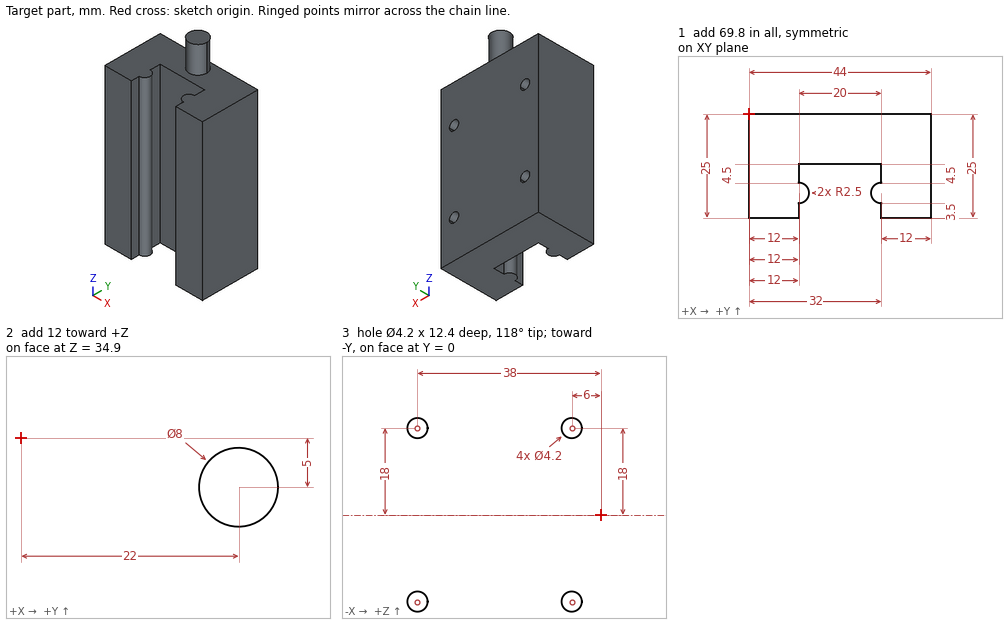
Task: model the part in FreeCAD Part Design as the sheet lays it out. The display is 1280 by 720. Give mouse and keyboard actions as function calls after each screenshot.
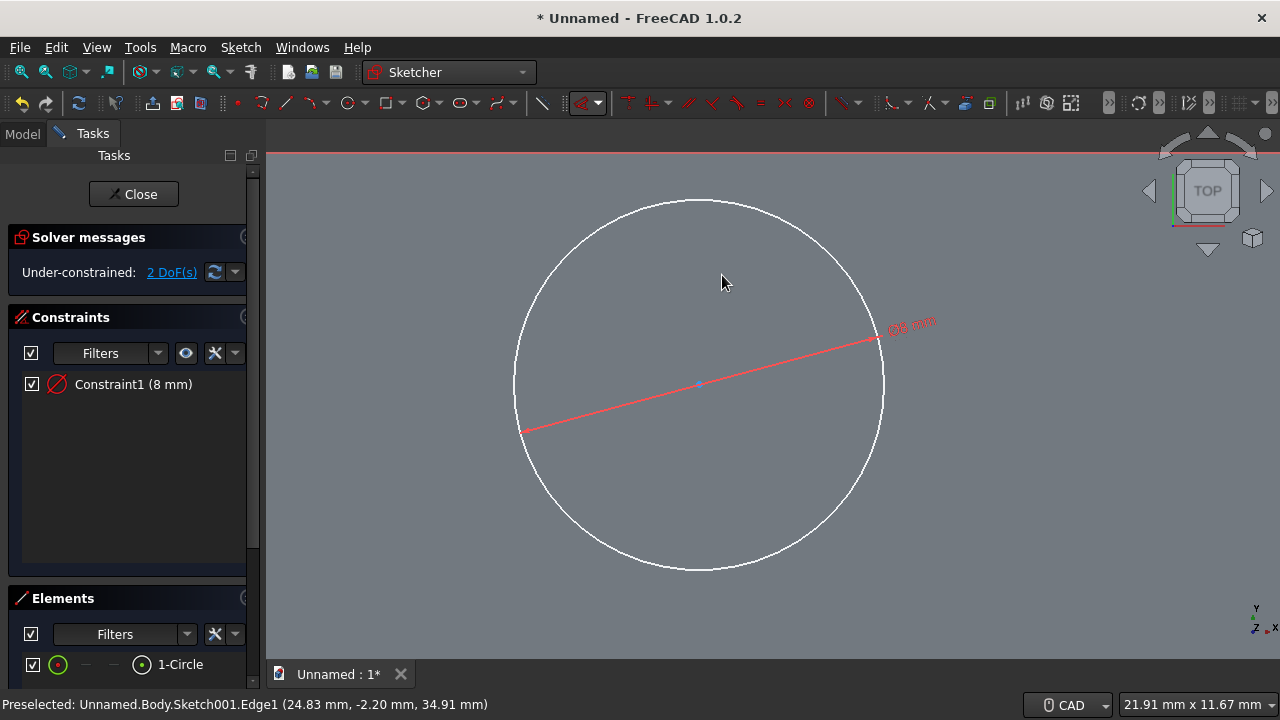
click(699, 385)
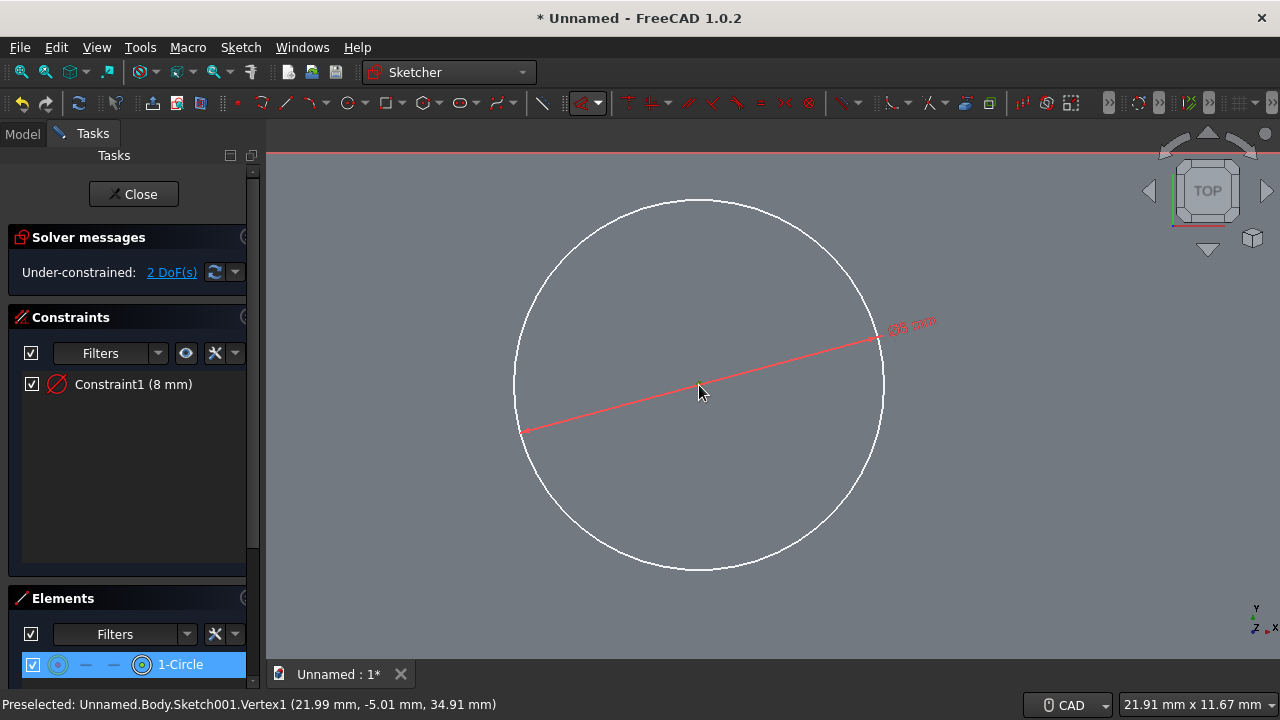
click(600, 104)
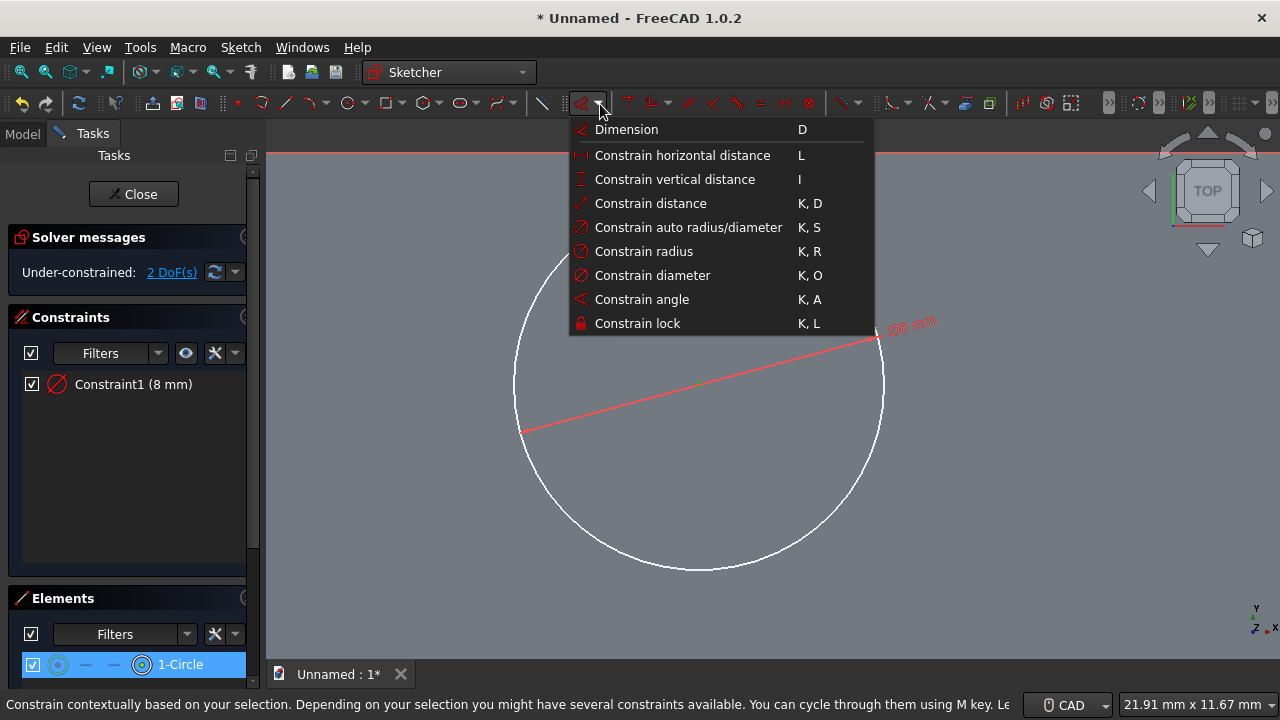
click(722, 179)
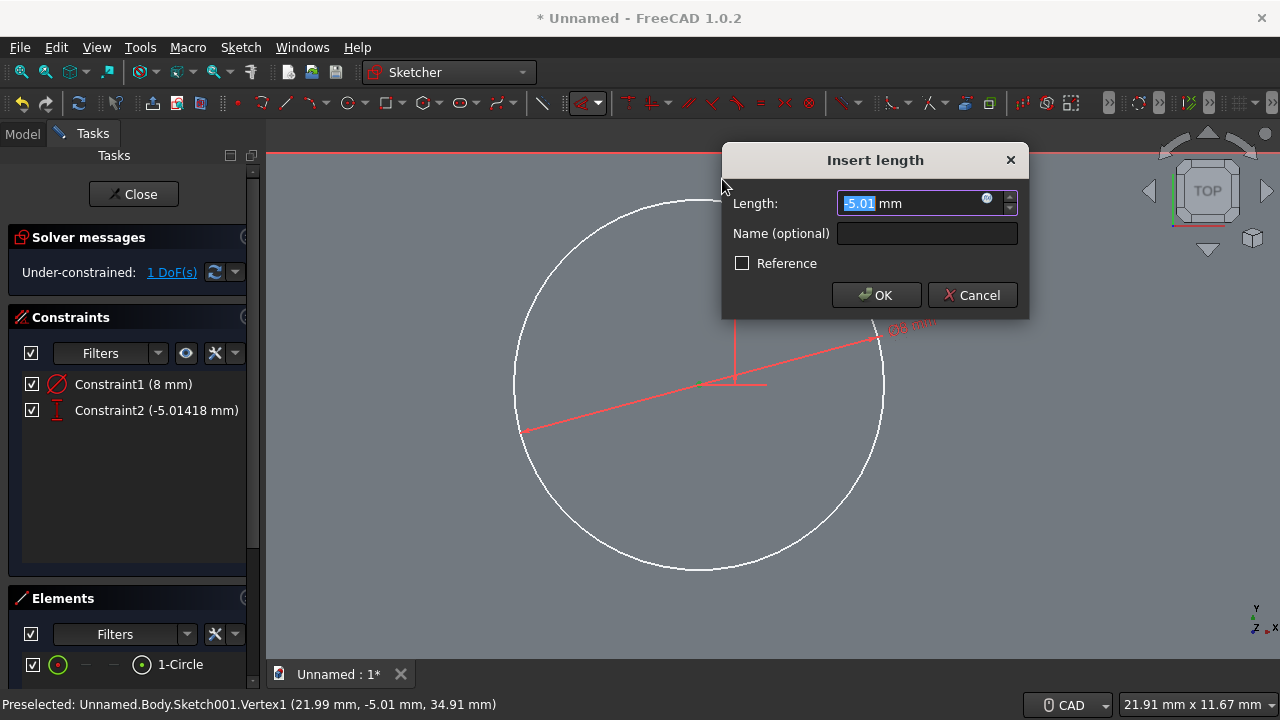
text(-5)
key(Return)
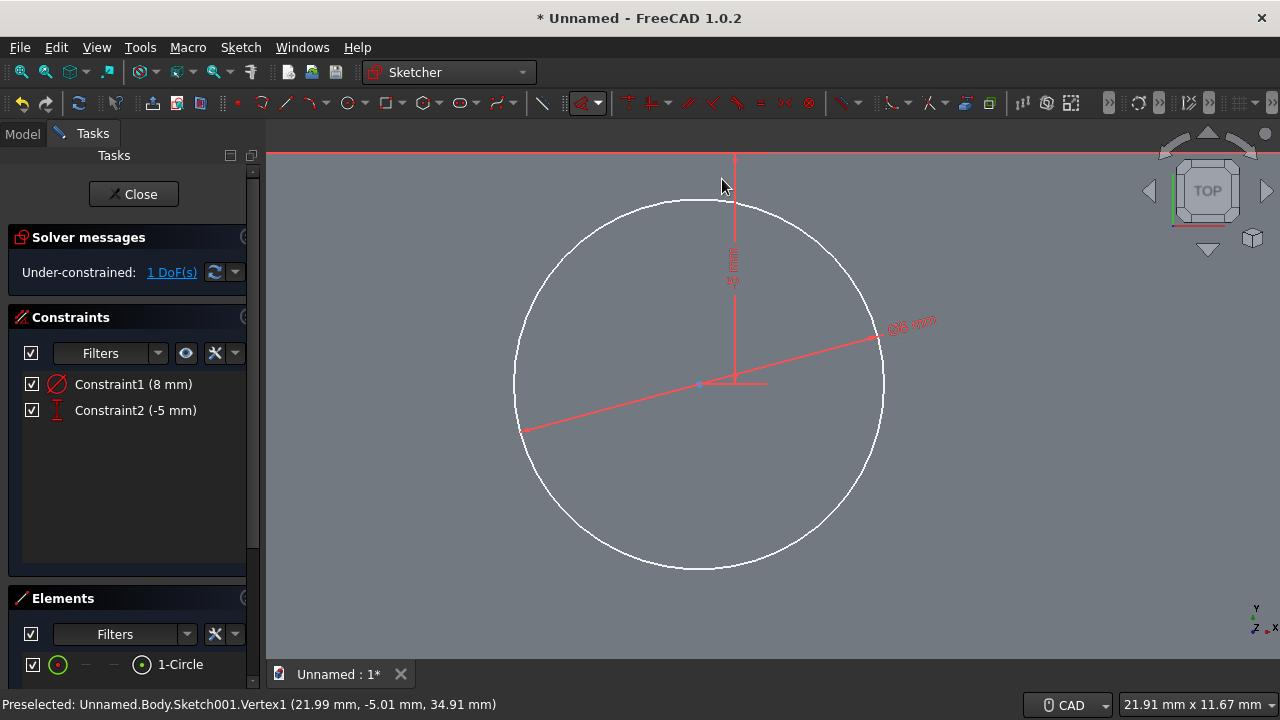
click(699, 384)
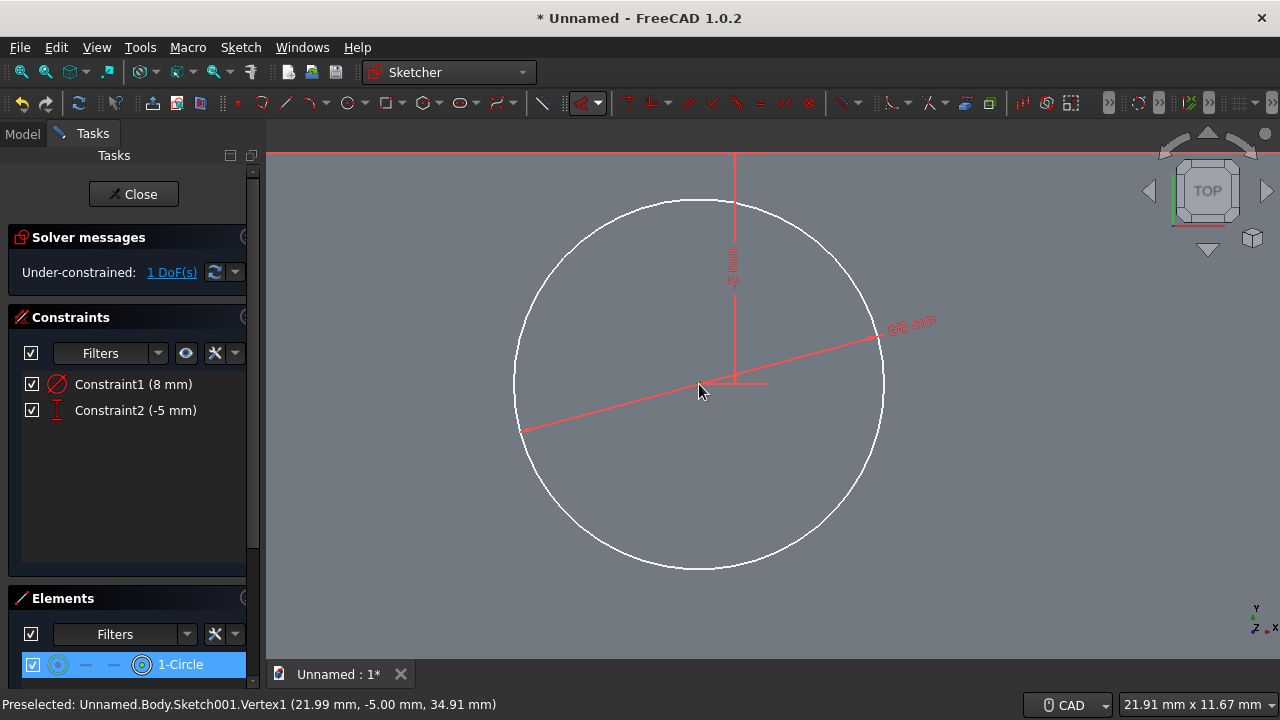
click(600, 104)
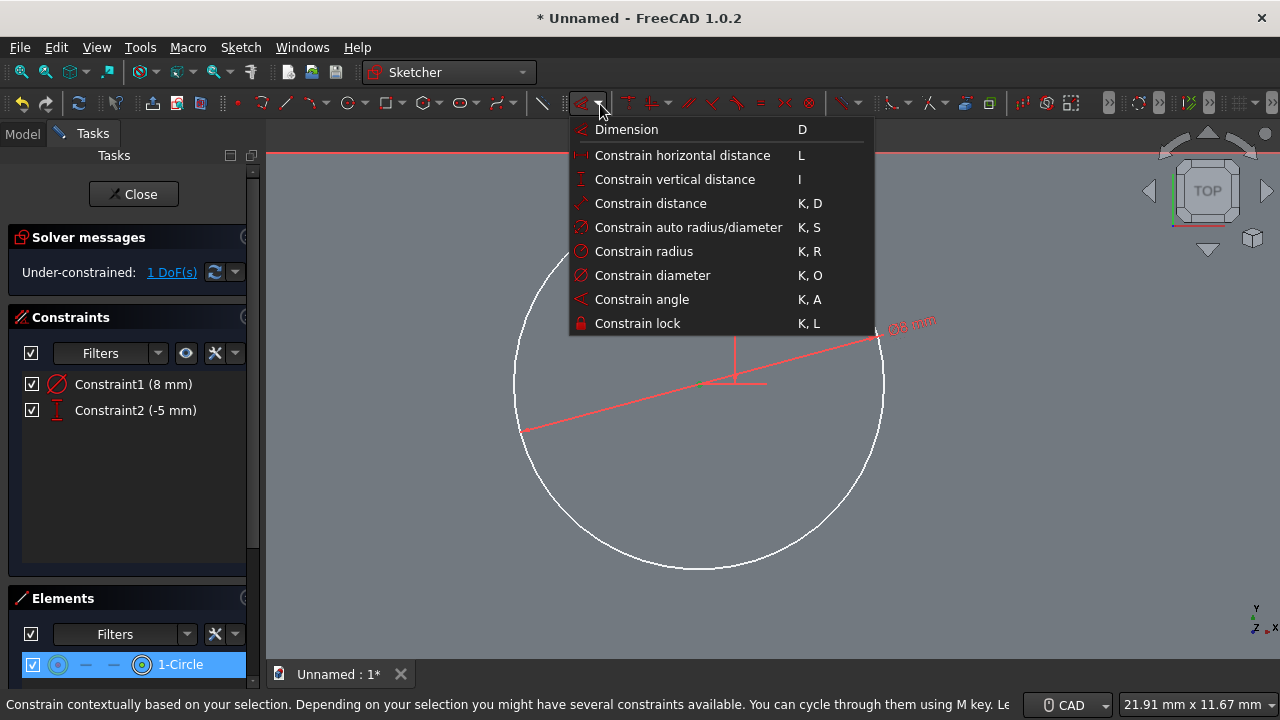
click(722, 155)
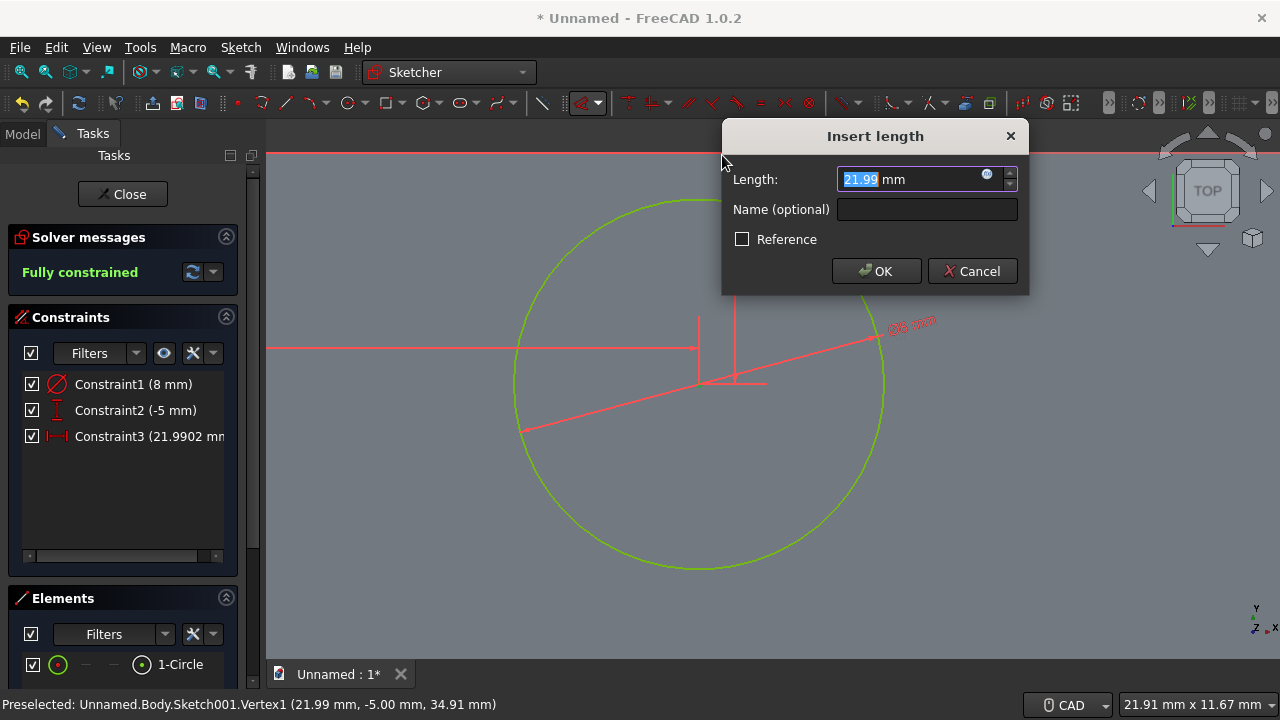
text(22)
key(Return)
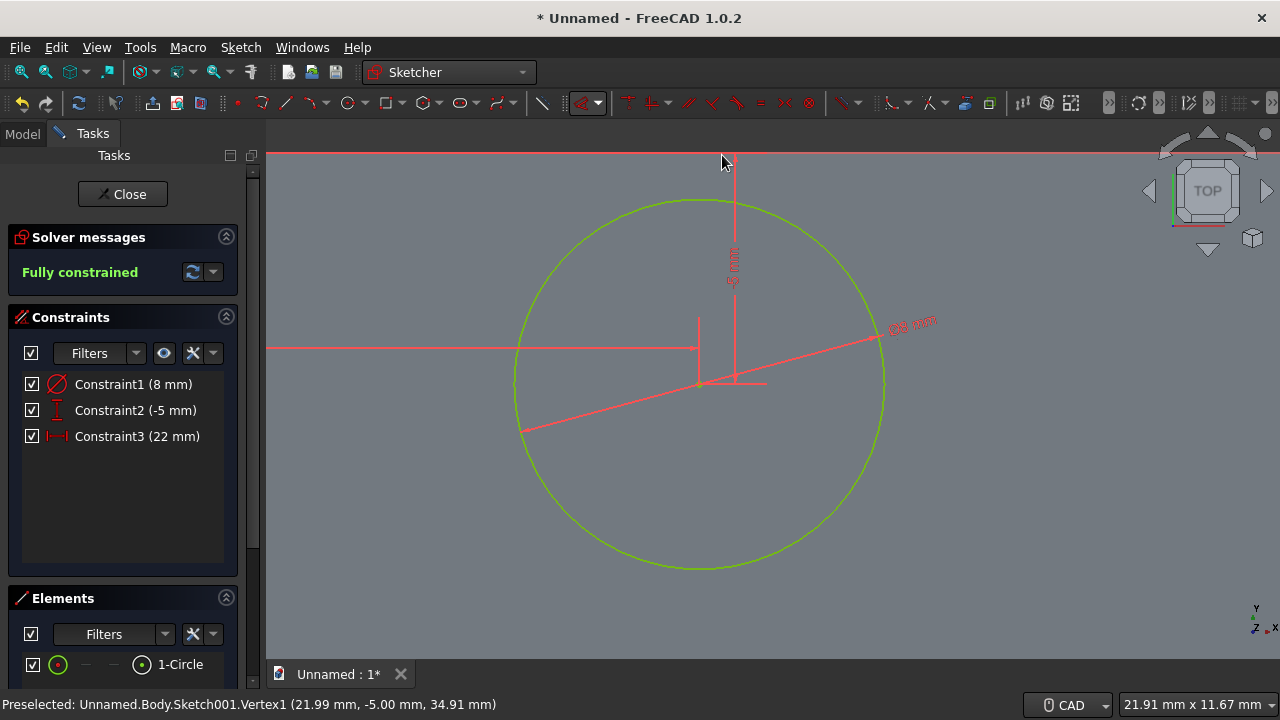
click(123, 194)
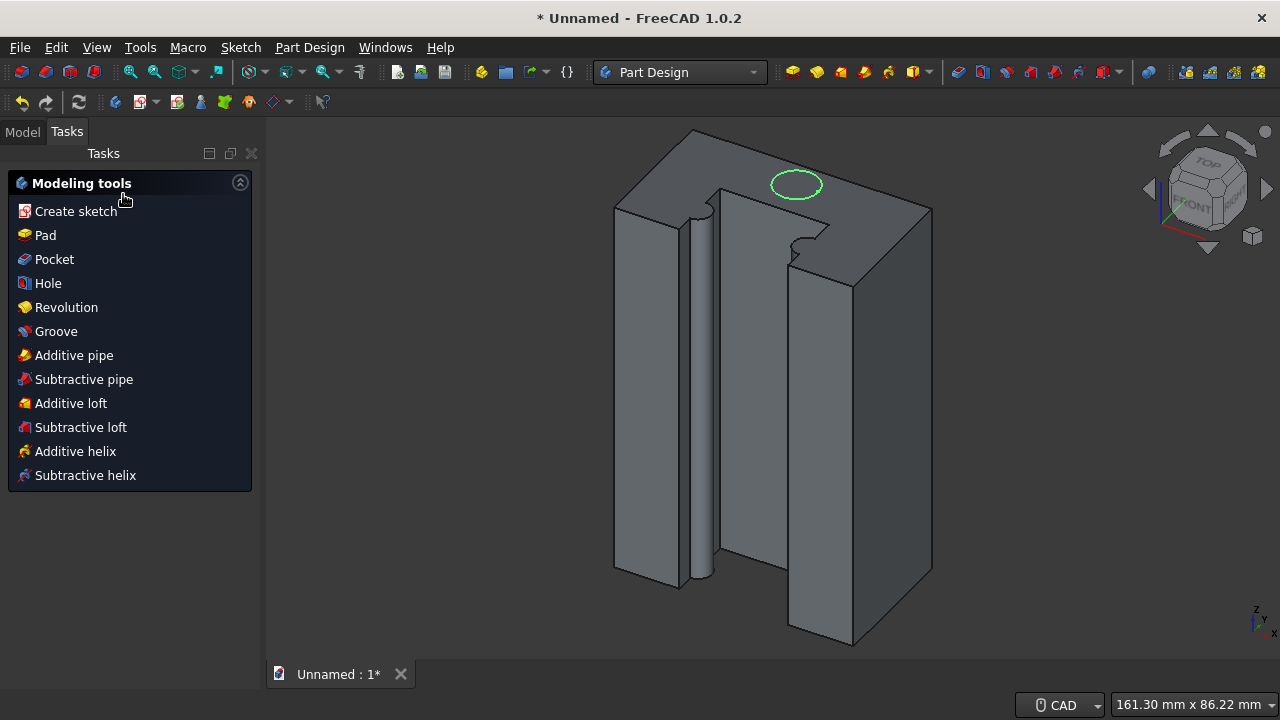
click(794, 72)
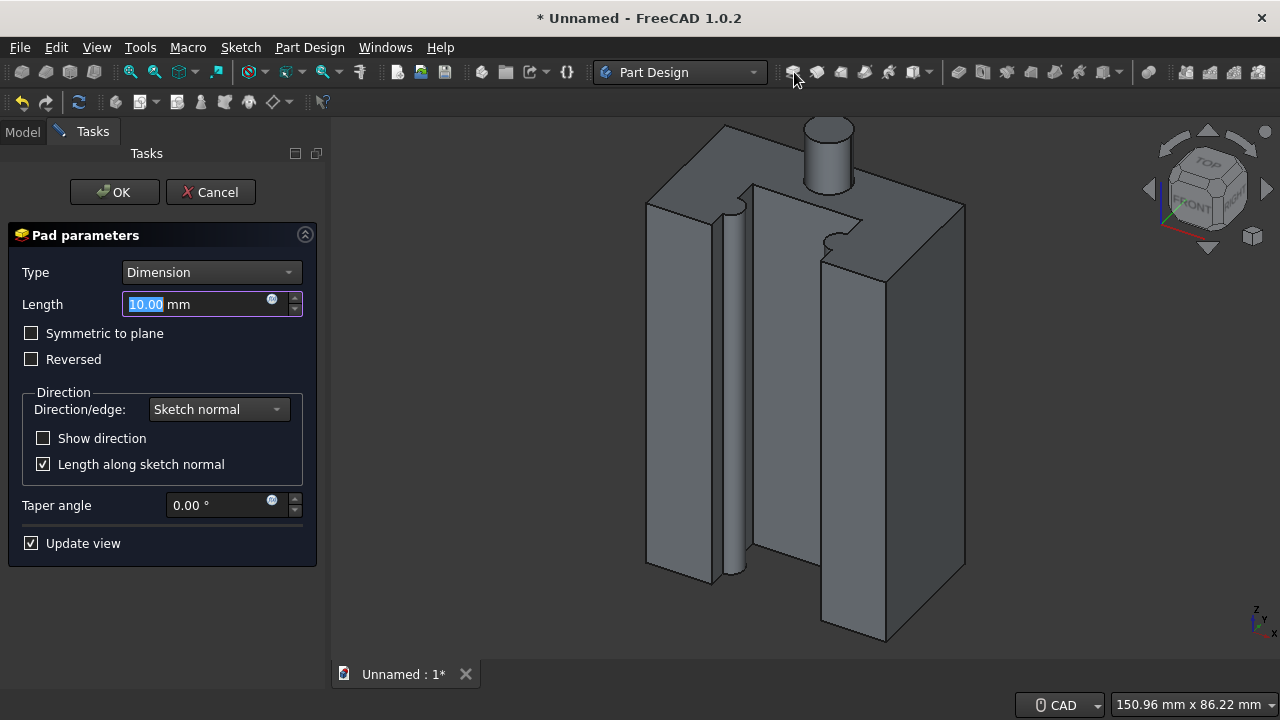
text(12)
key(Tab)